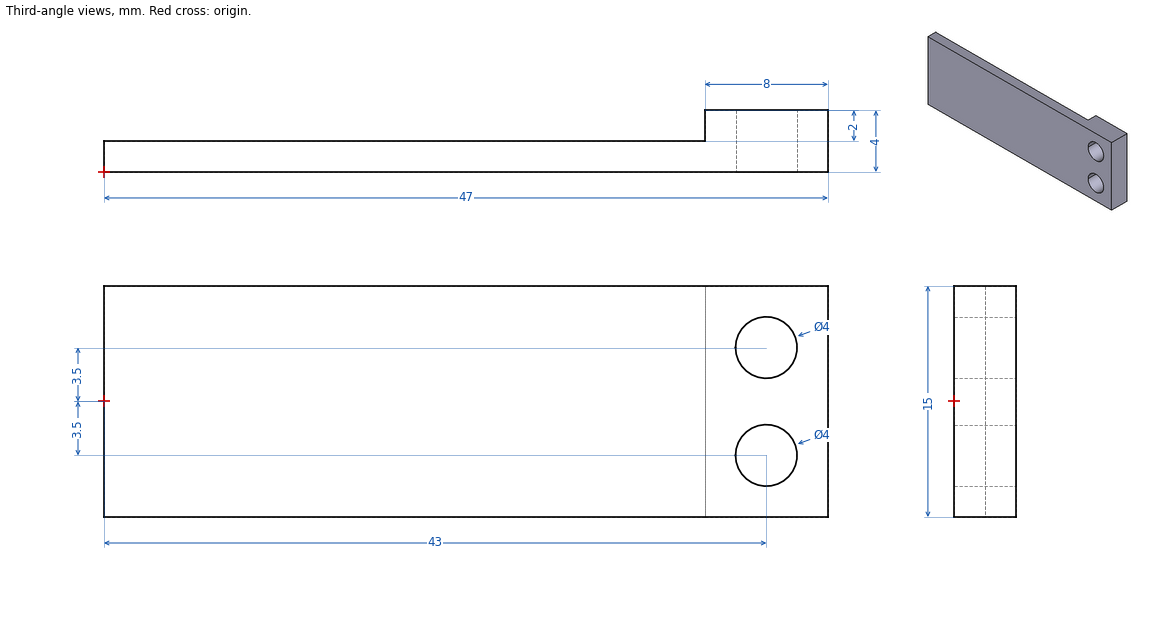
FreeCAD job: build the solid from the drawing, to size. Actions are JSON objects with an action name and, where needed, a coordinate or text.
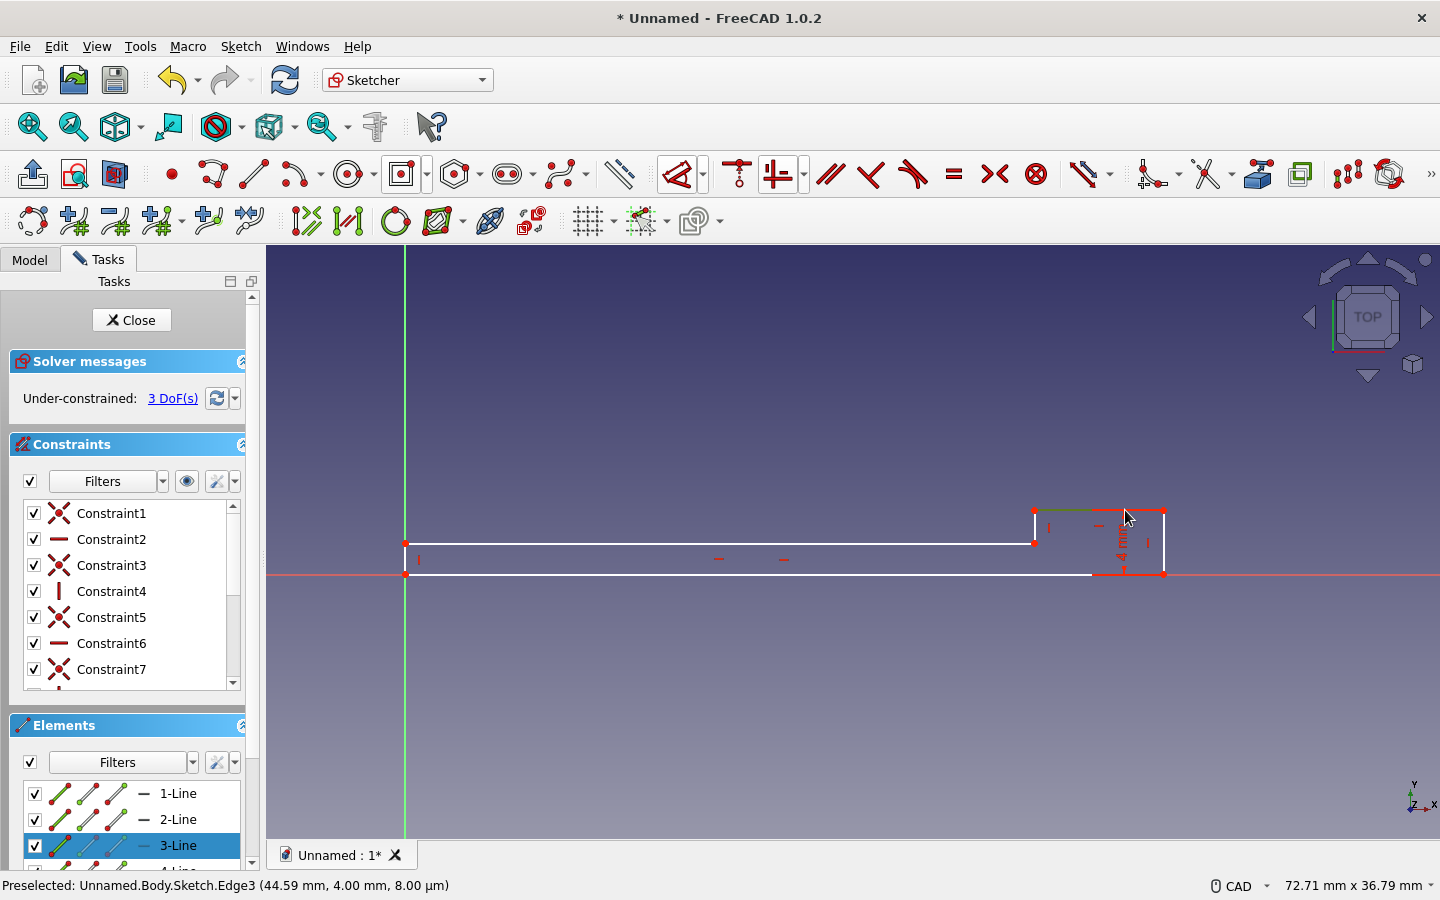
{"action": "left_click", "coordinate": [702, 174]}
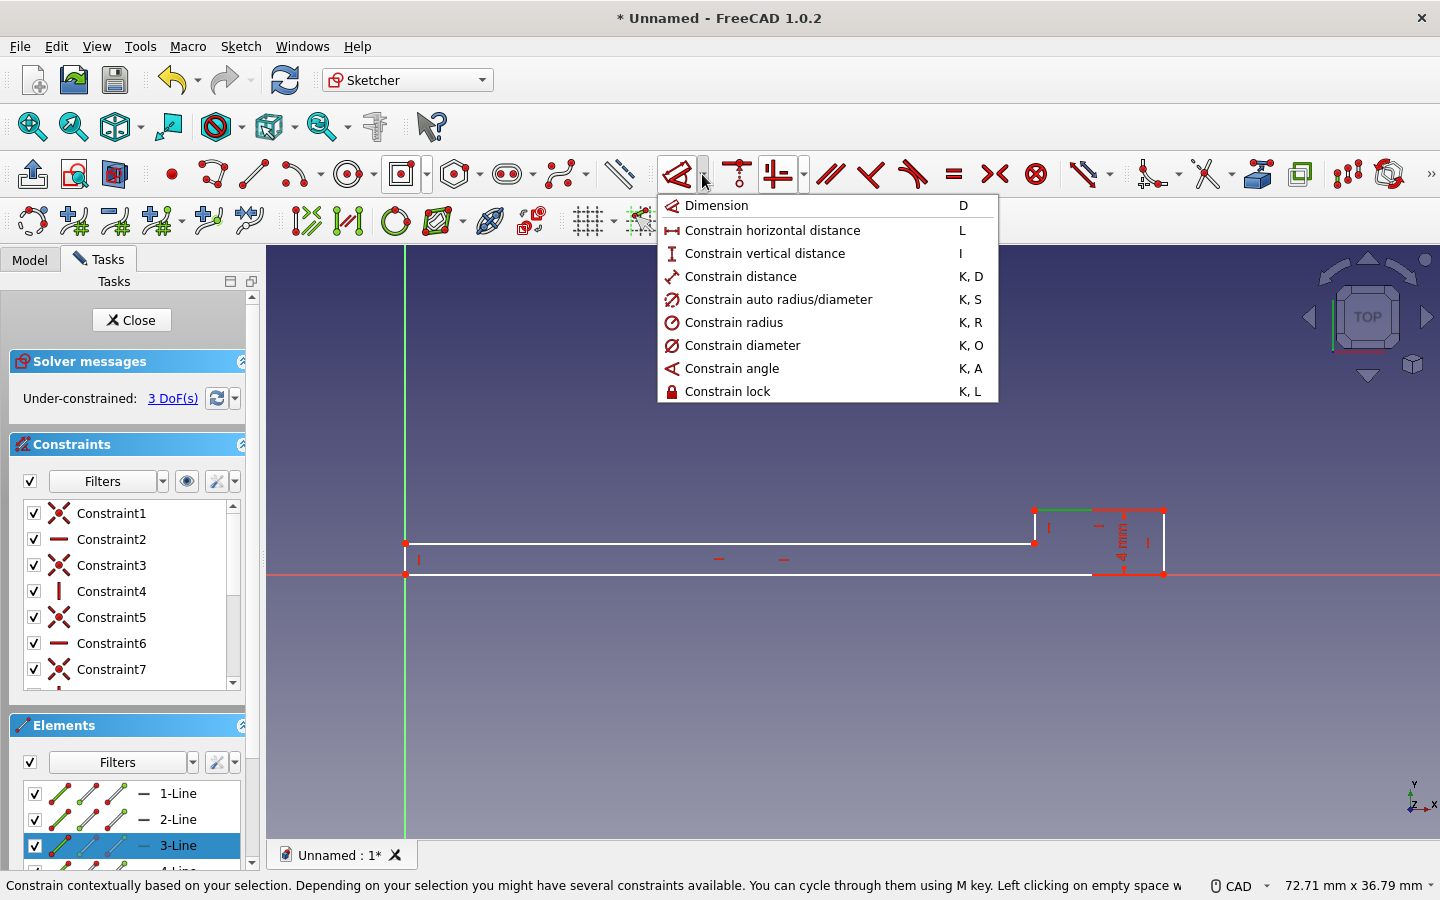
{"action": "left_click", "coordinate": [828, 230]}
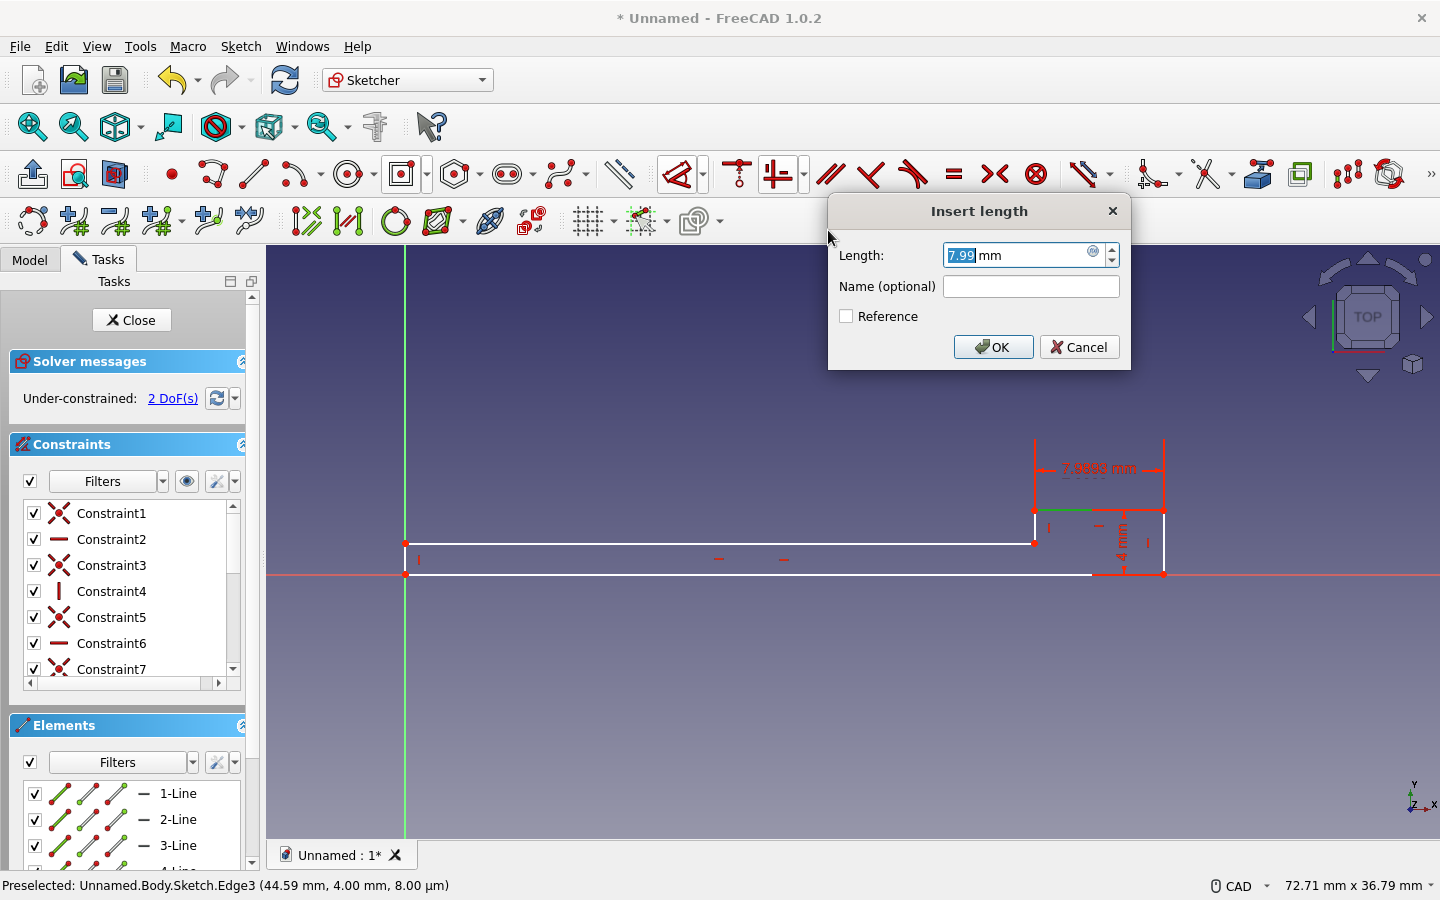
{"action": "type", "text": "8"}
{"action": "key", "text": "Return"}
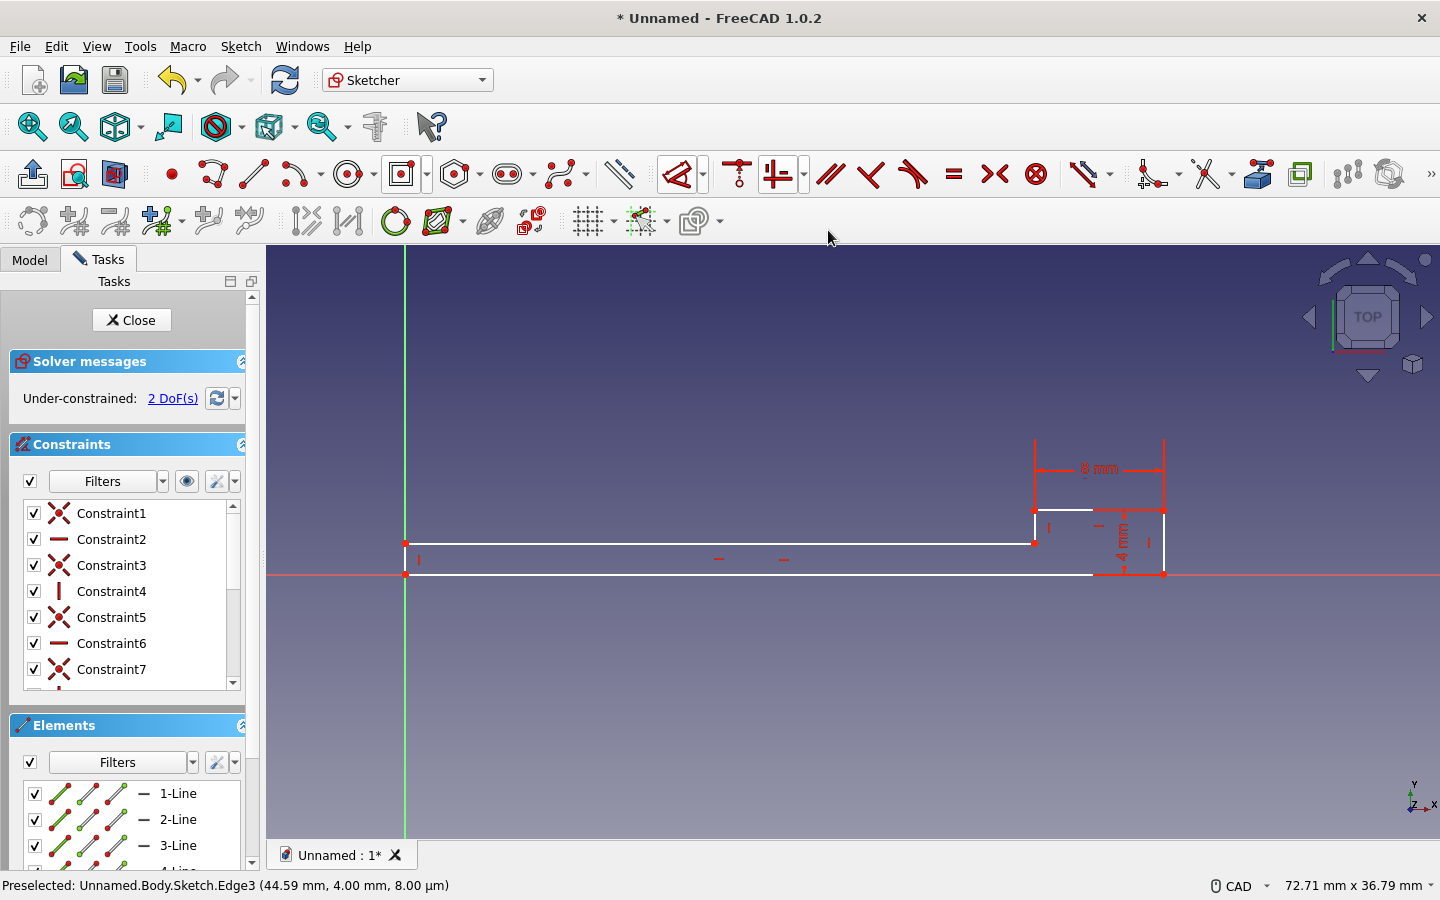
{"action": "scroll", "coordinate": [1035, 520], "scroll_direction": "up", "scroll_amount": 2}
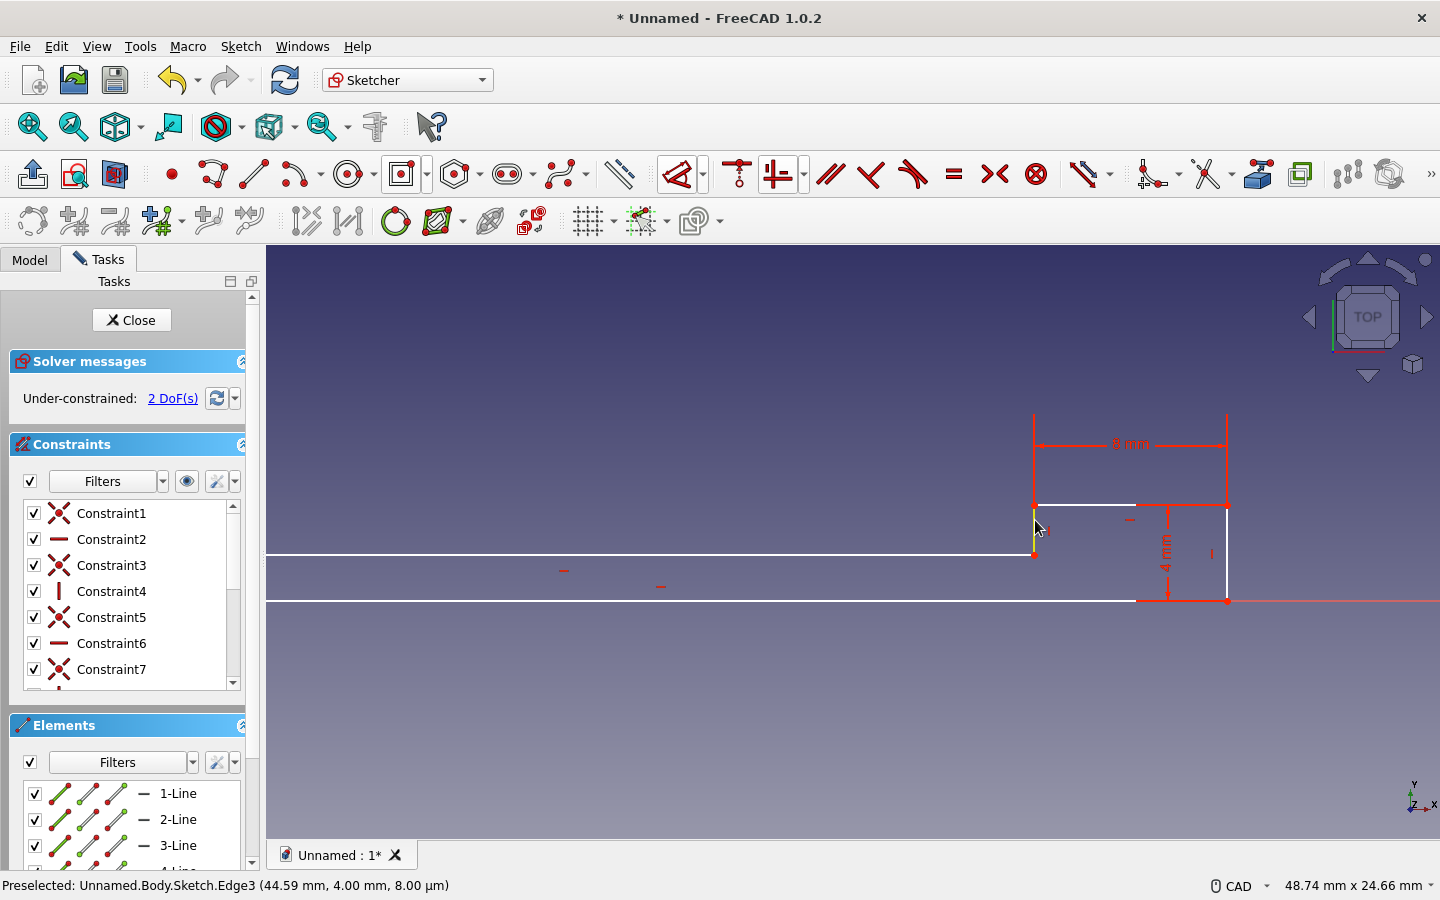
{"action": "left_click", "coordinate": [1034, 520]}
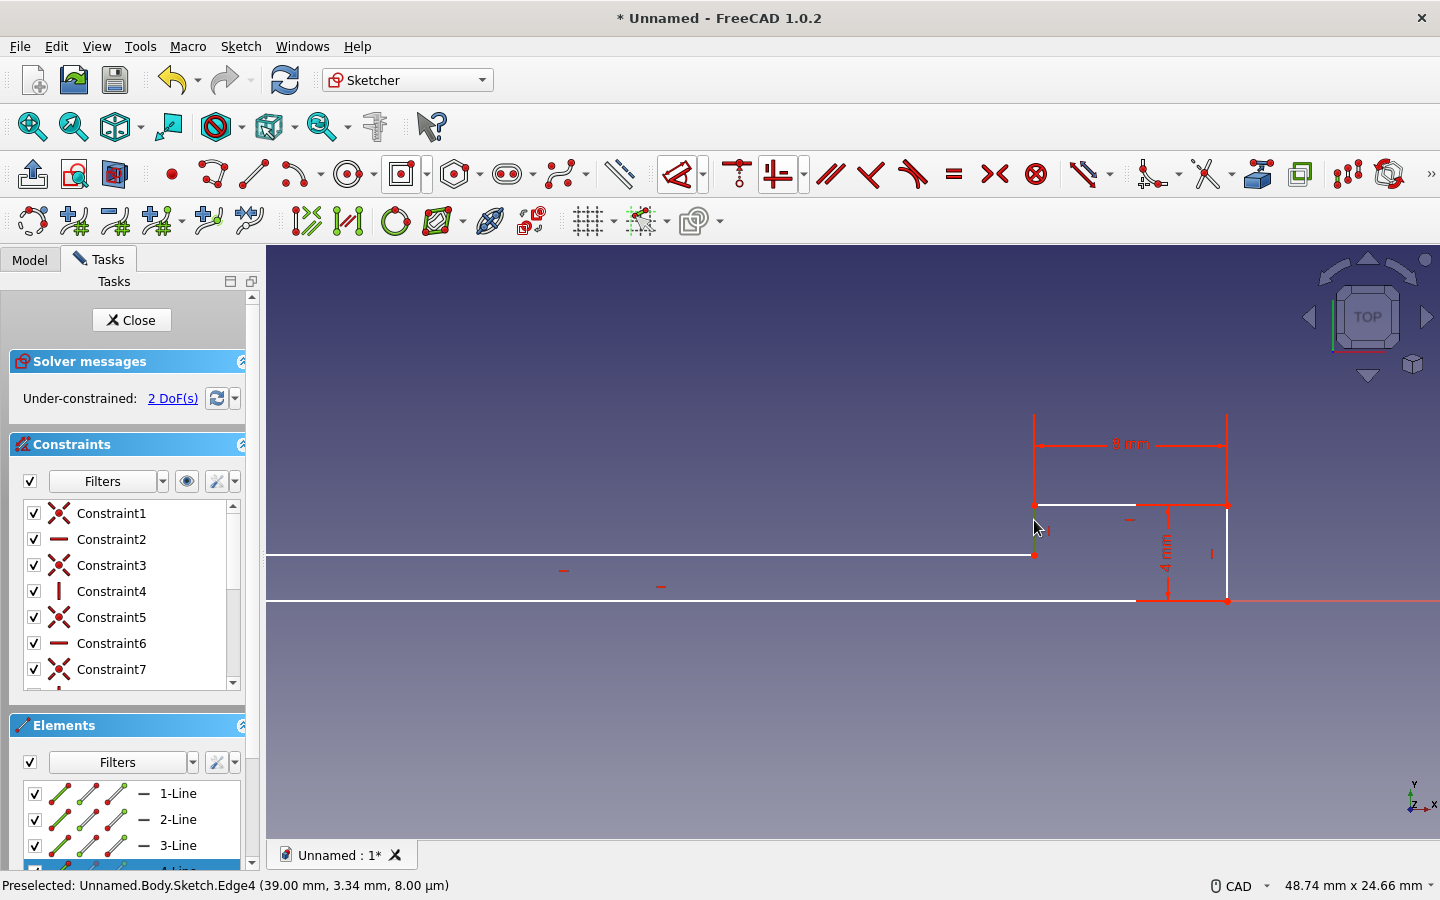
{"action": "key", "text": "i"}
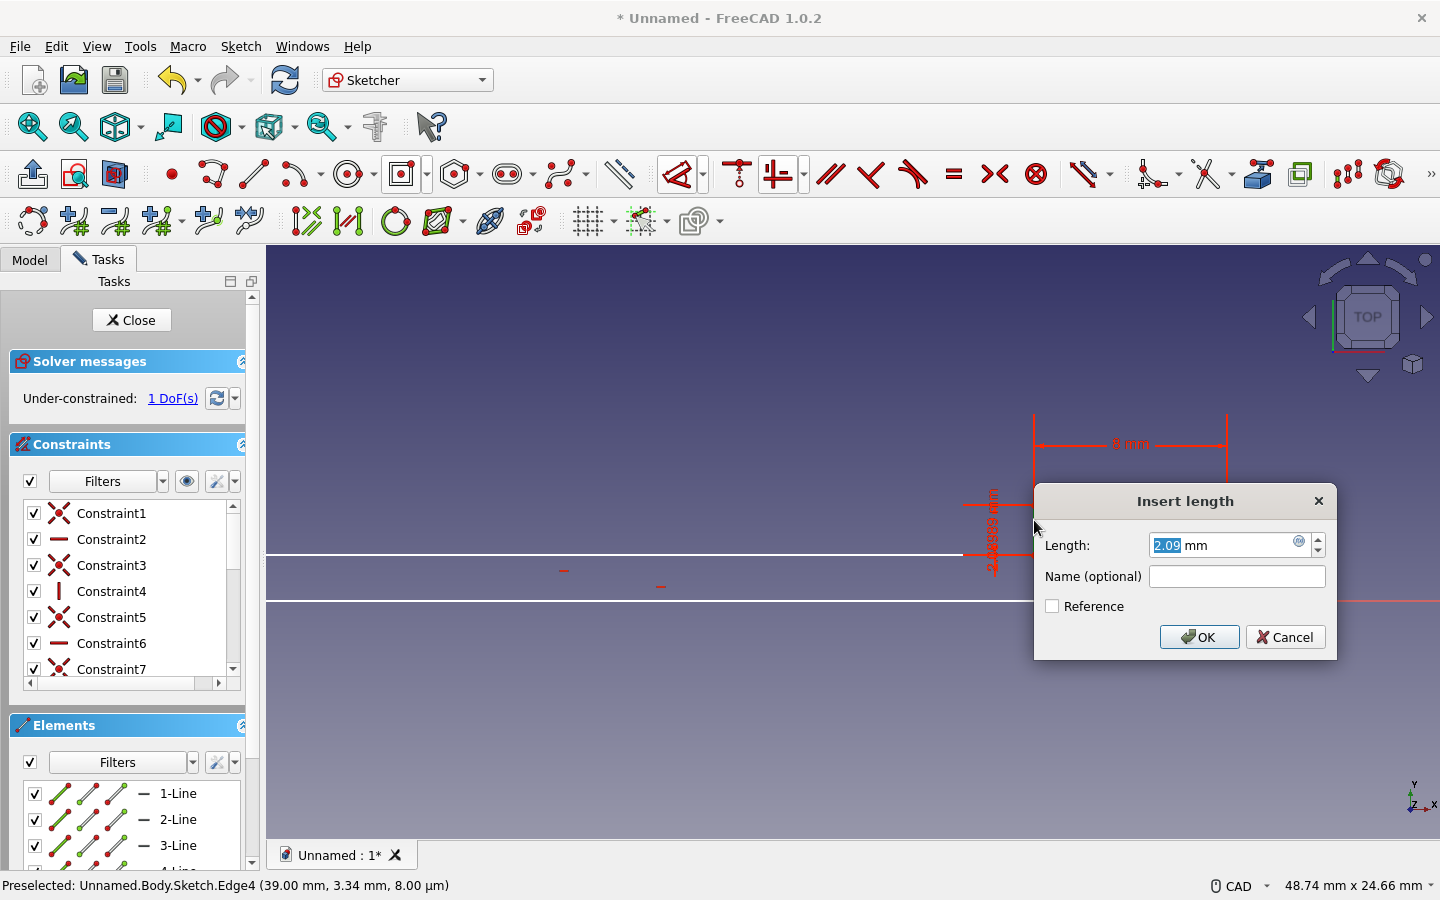
{"action": "type", "text": "2"}
{"action": "key", "text": "Return"}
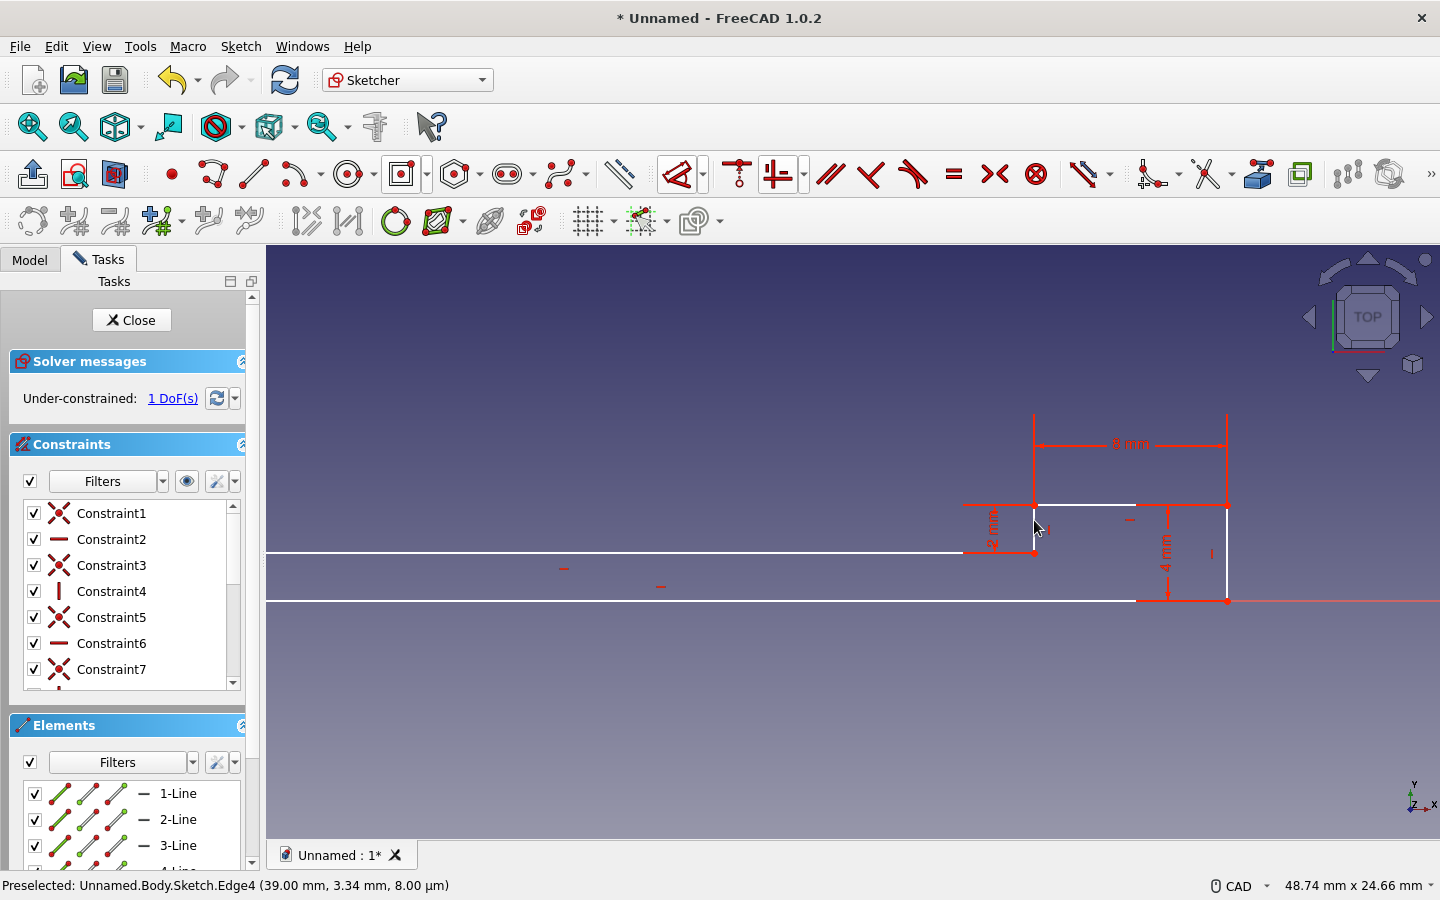
{"action": "left_click", "coordinate": [435, 601]}